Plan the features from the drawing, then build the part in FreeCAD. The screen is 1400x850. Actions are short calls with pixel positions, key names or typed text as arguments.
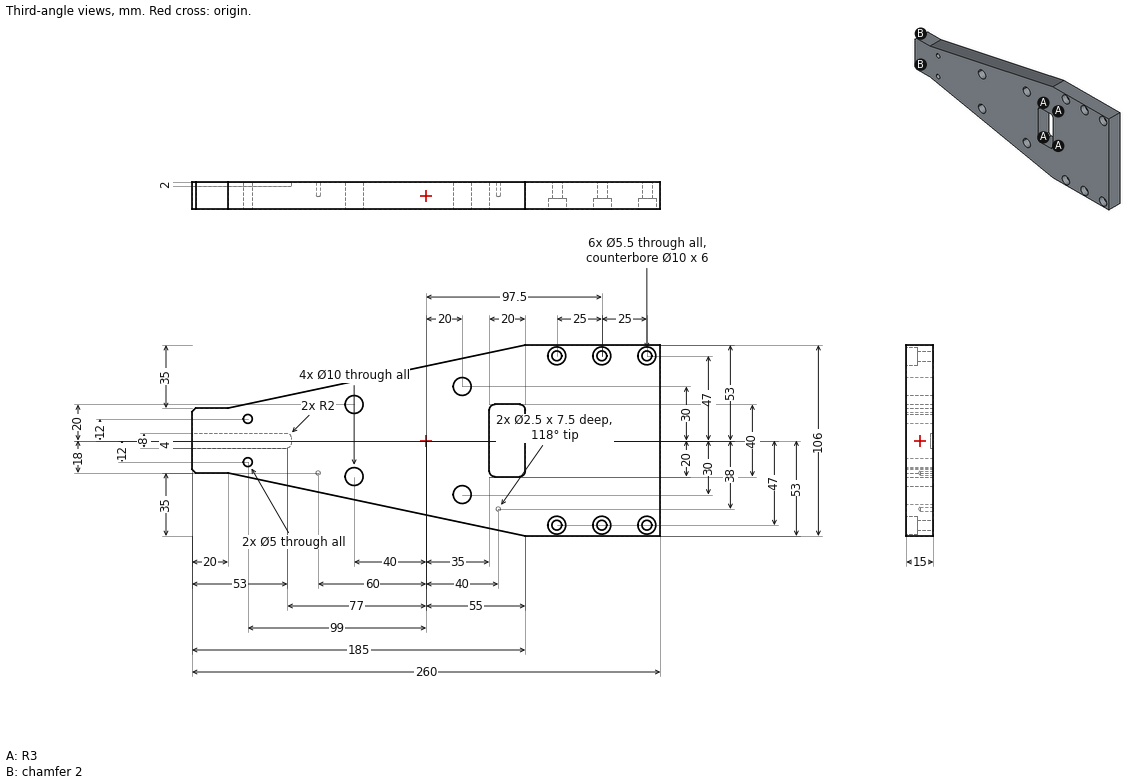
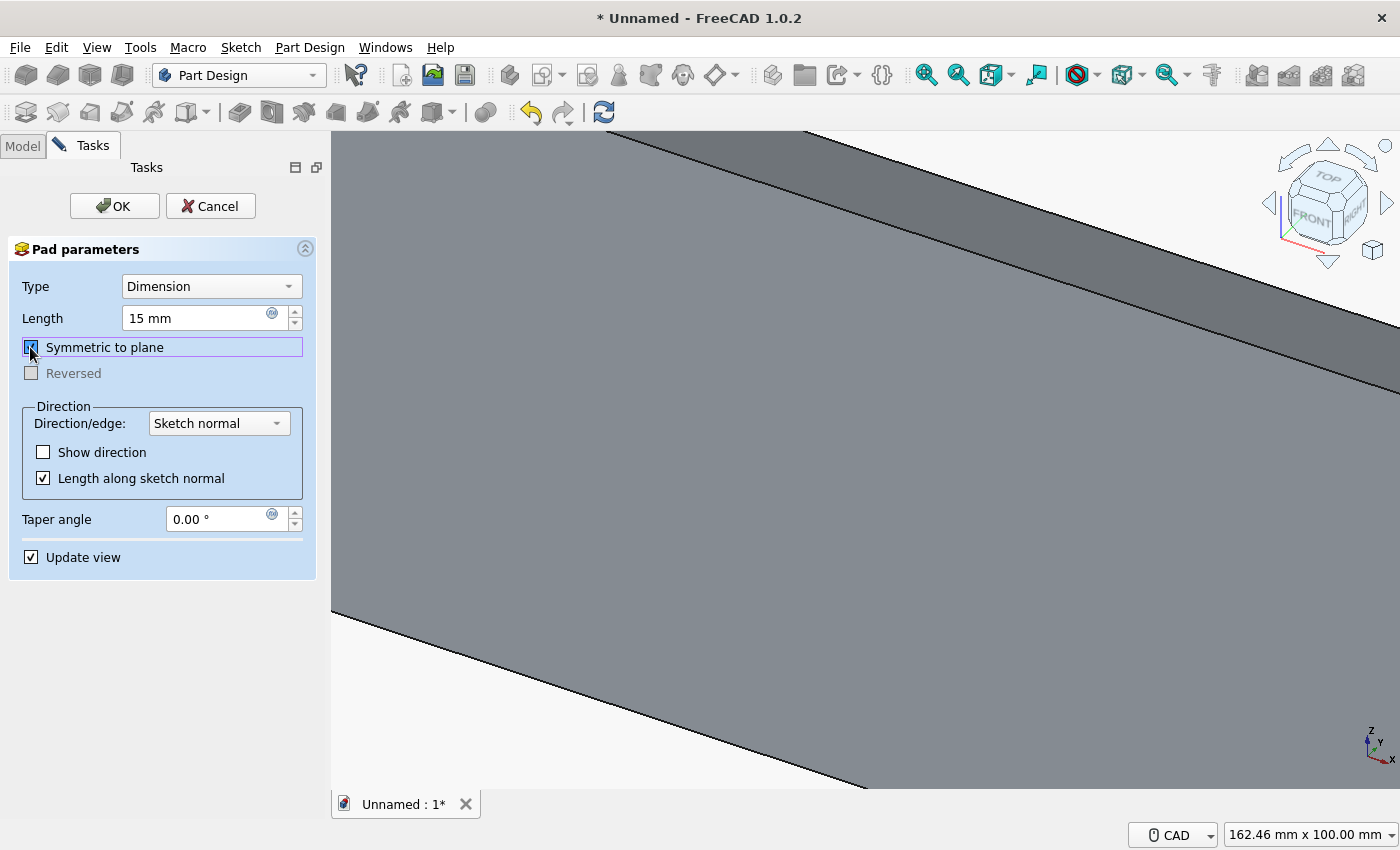
click(115, 206)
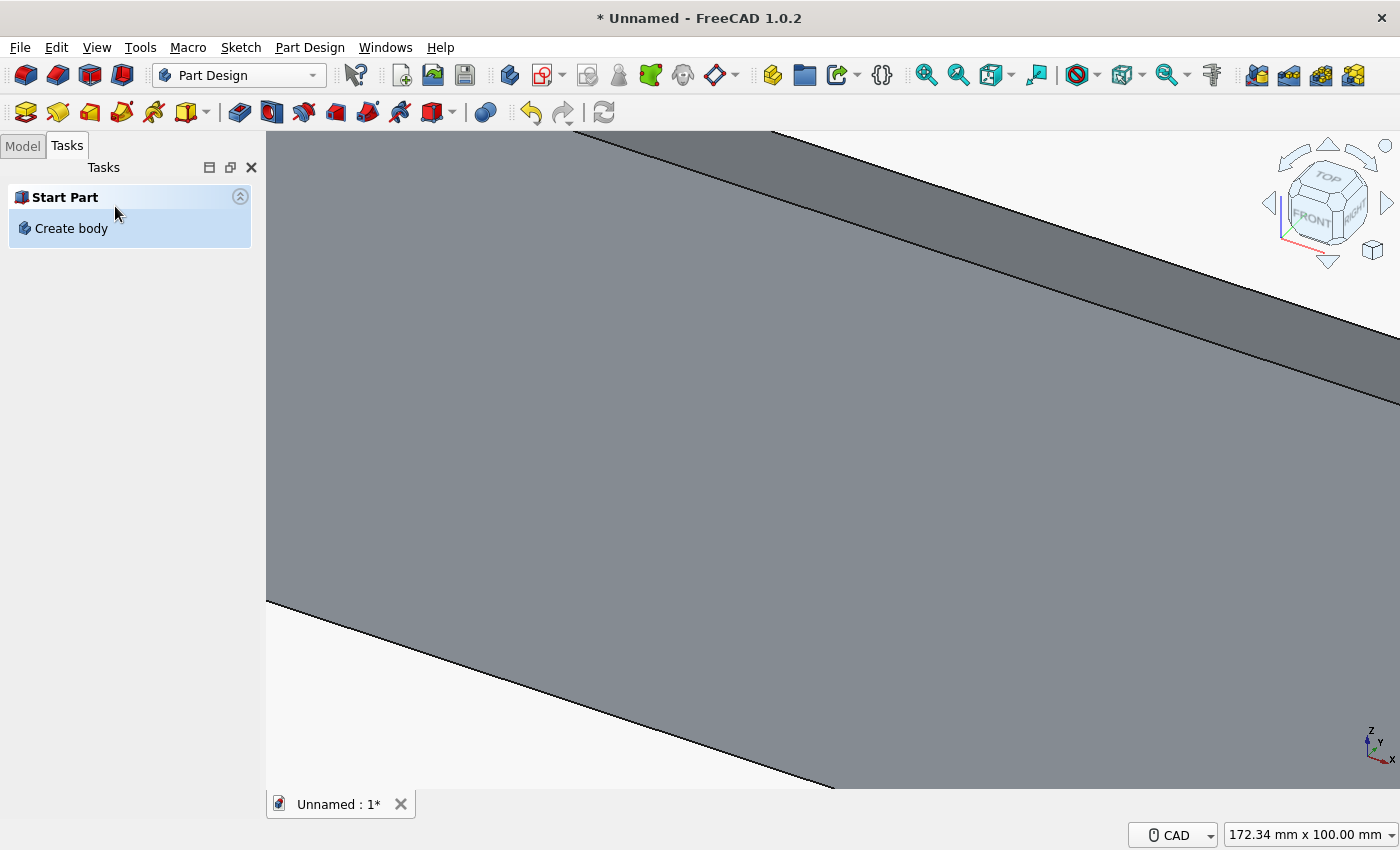
key(v)
key(f)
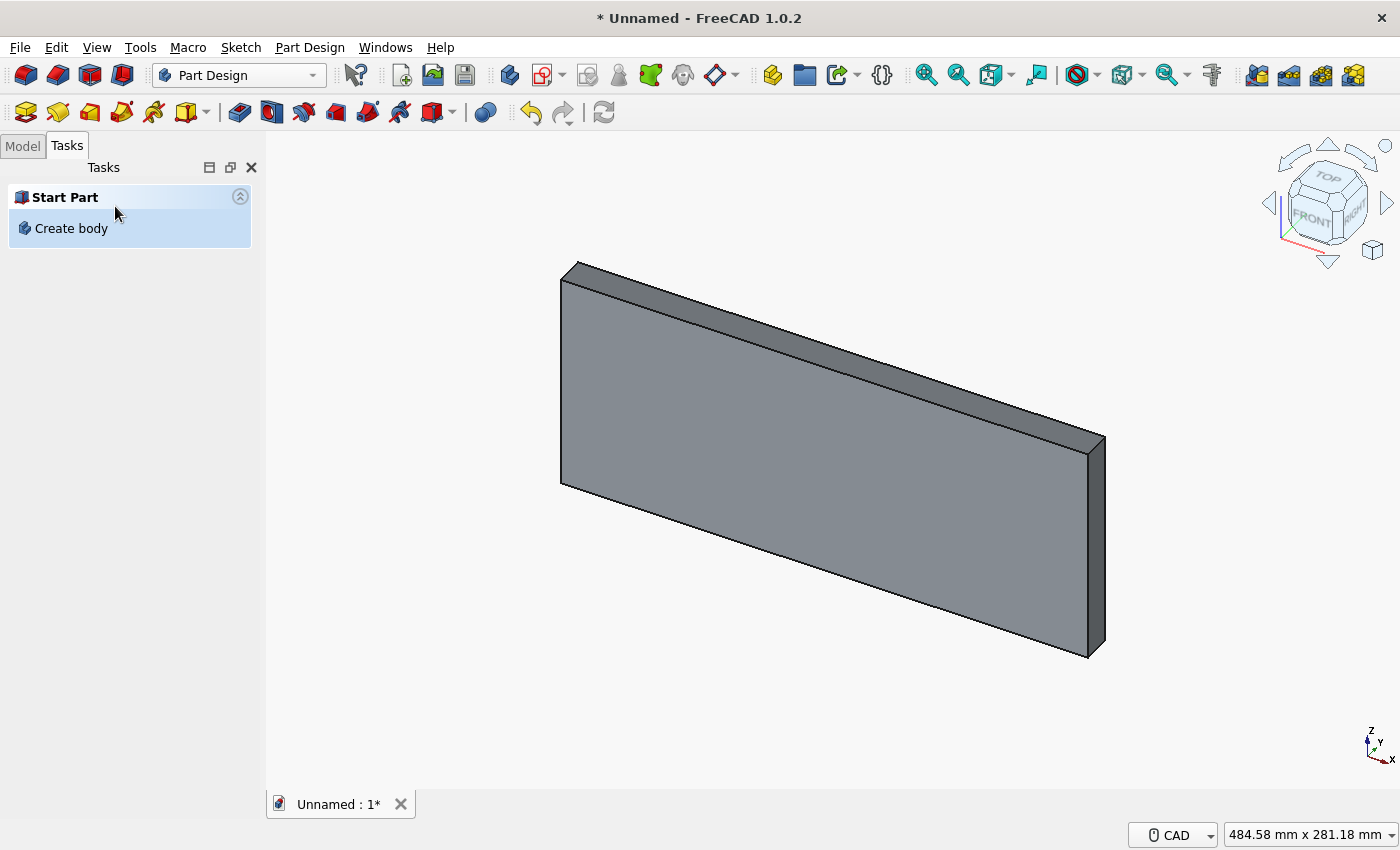
key(4)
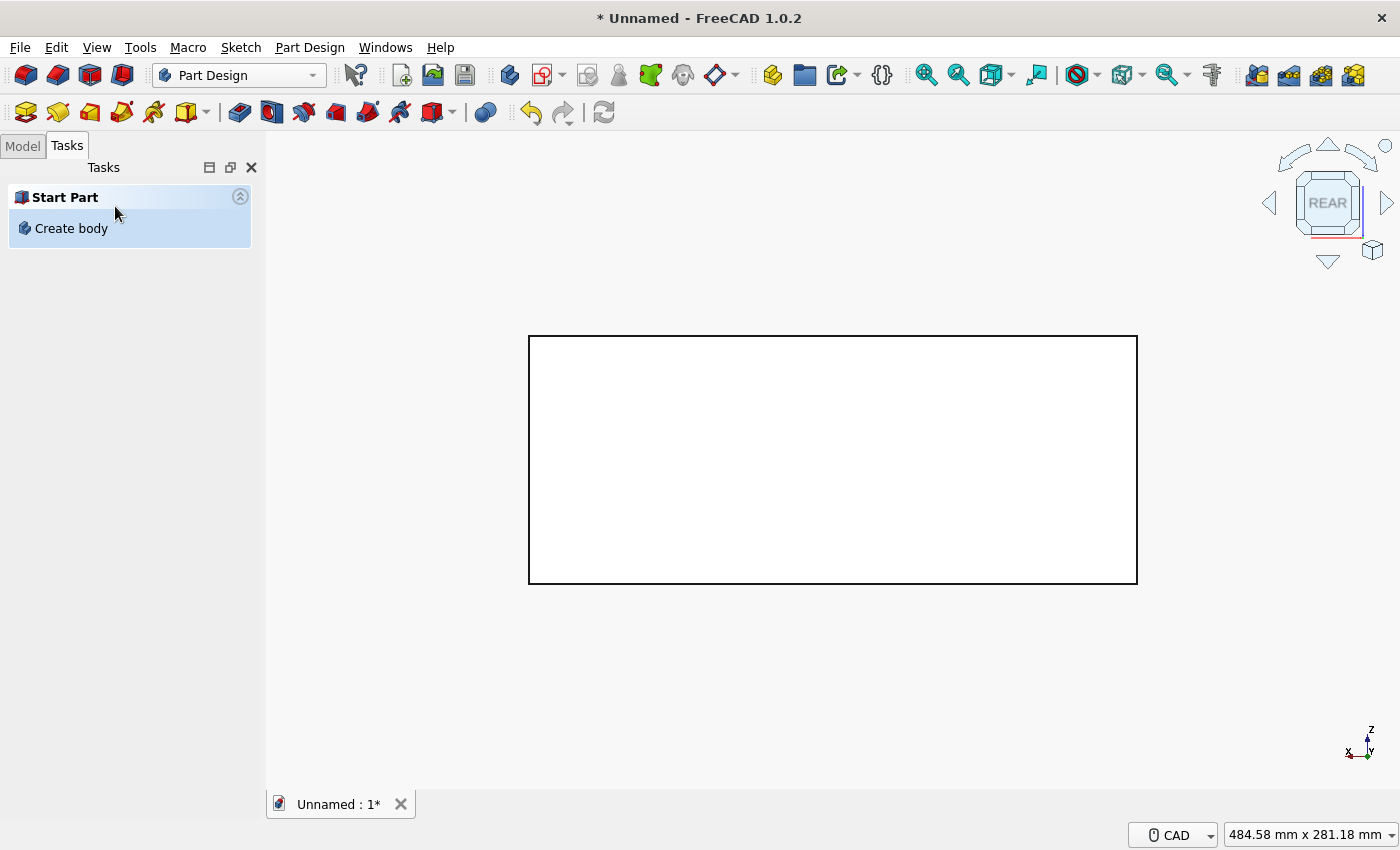
click(659, 459)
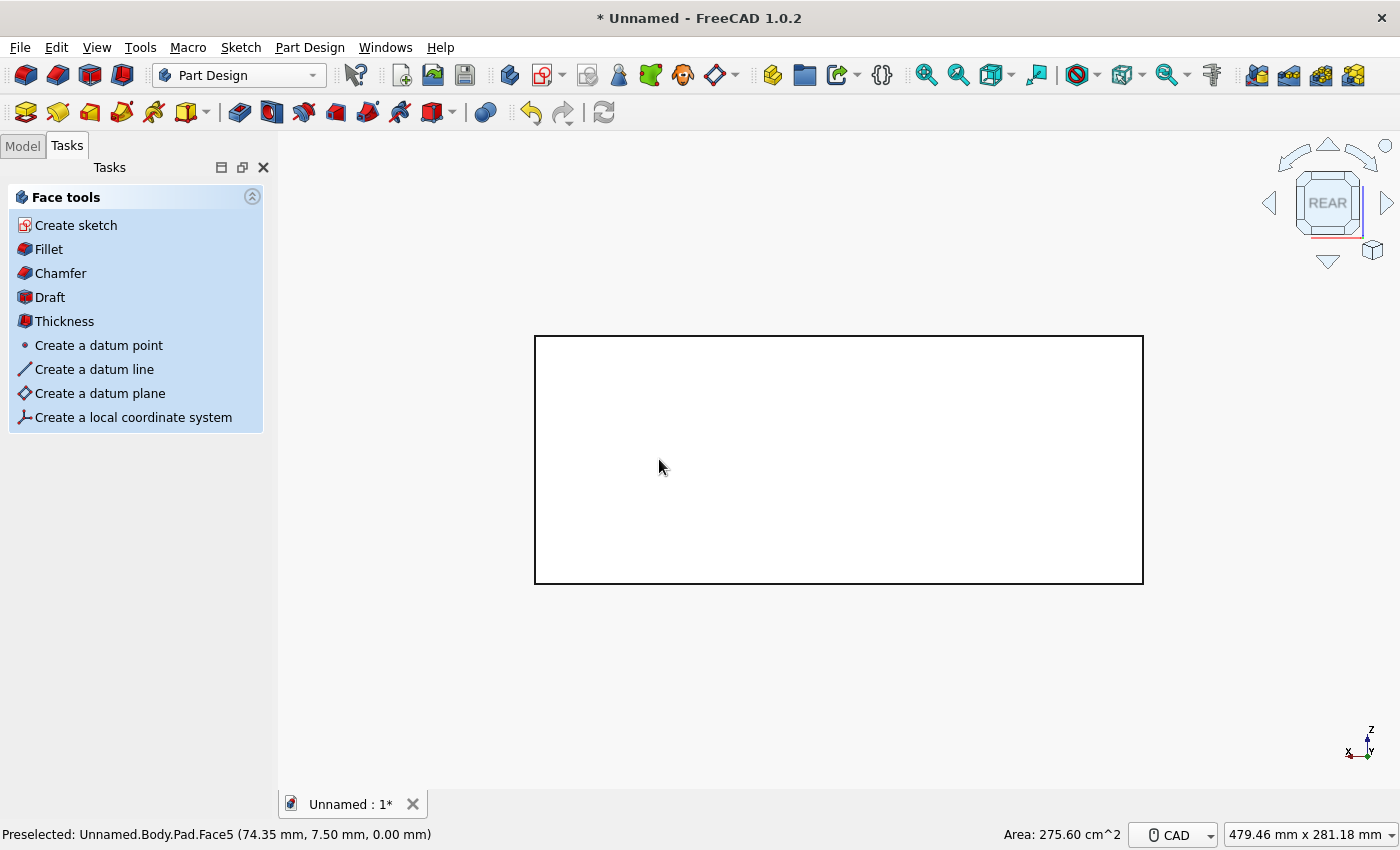
click(542, 76)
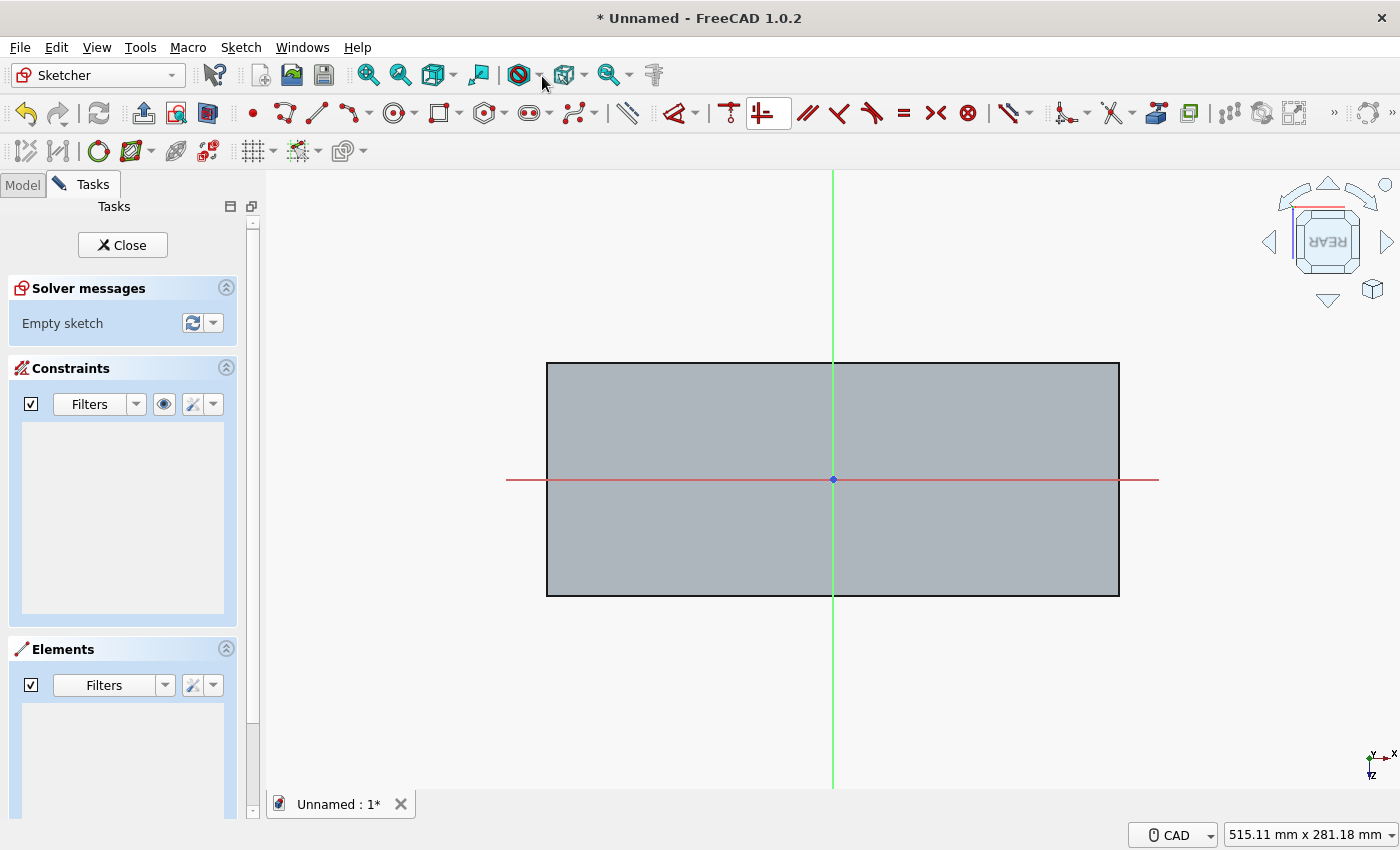
scroll(722, 480, up, 2)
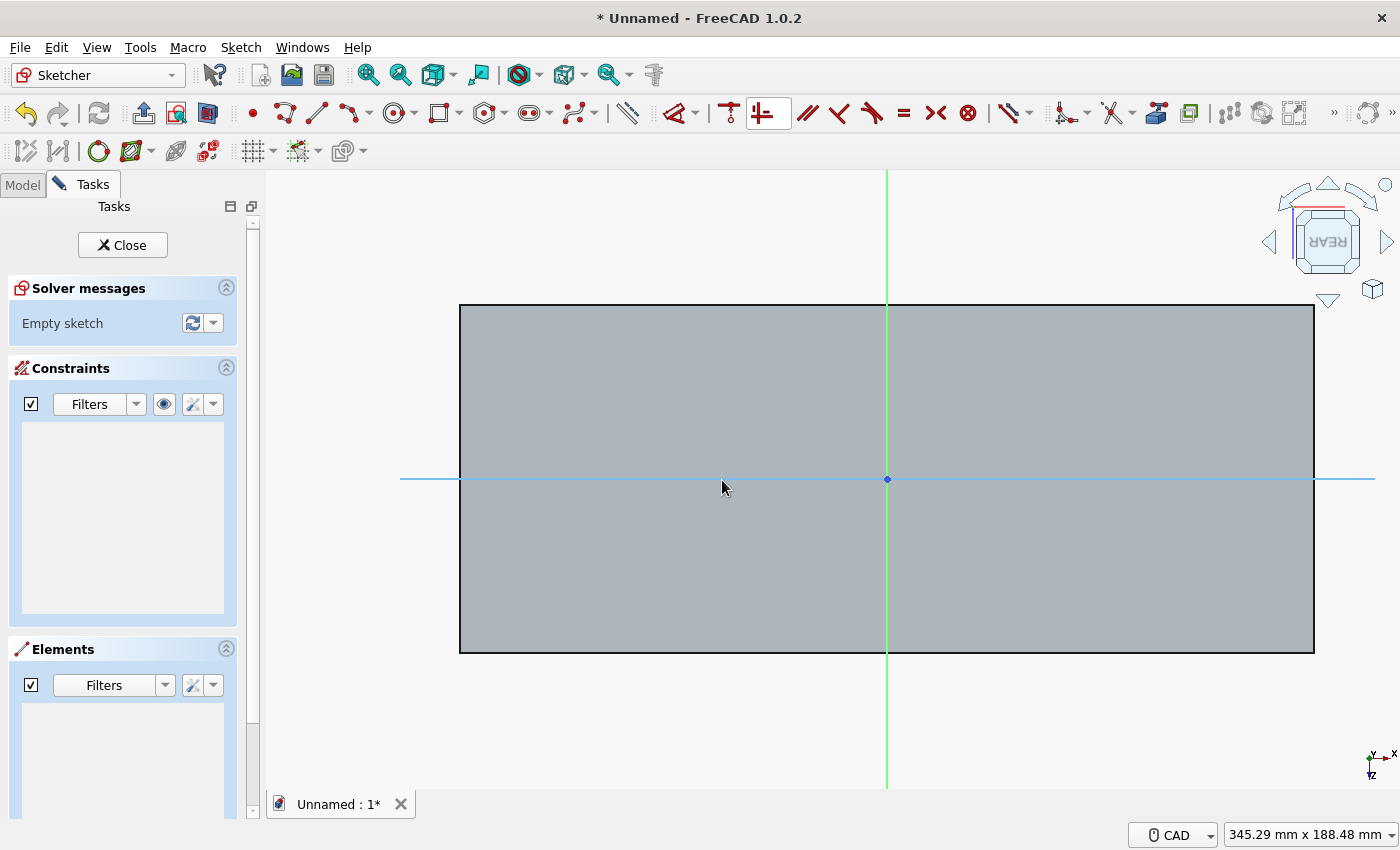
click(286, 114)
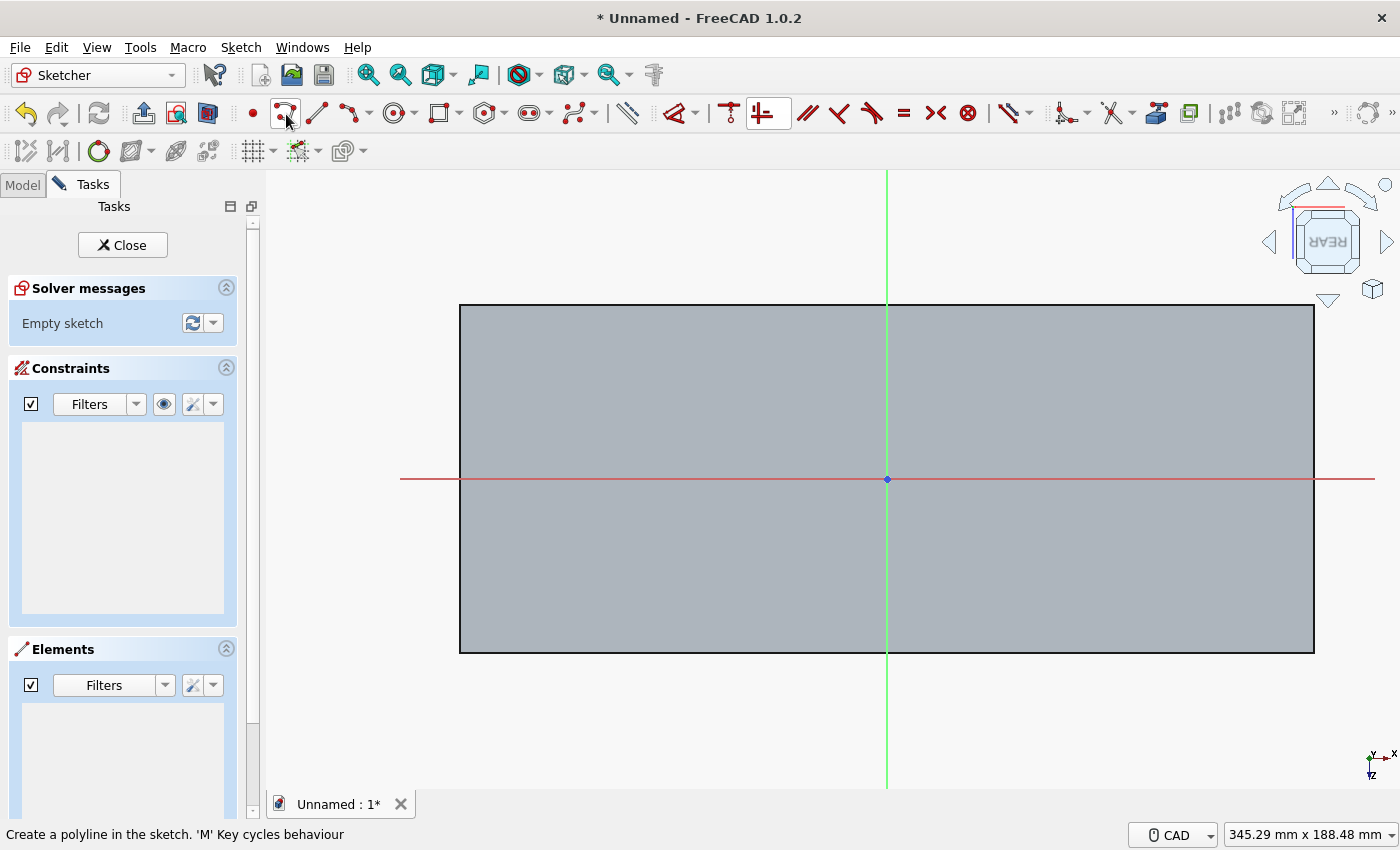
click(1068, 305)
click(460, 305)
click(460, 420)
click(526, 420)
click(1068, 306)